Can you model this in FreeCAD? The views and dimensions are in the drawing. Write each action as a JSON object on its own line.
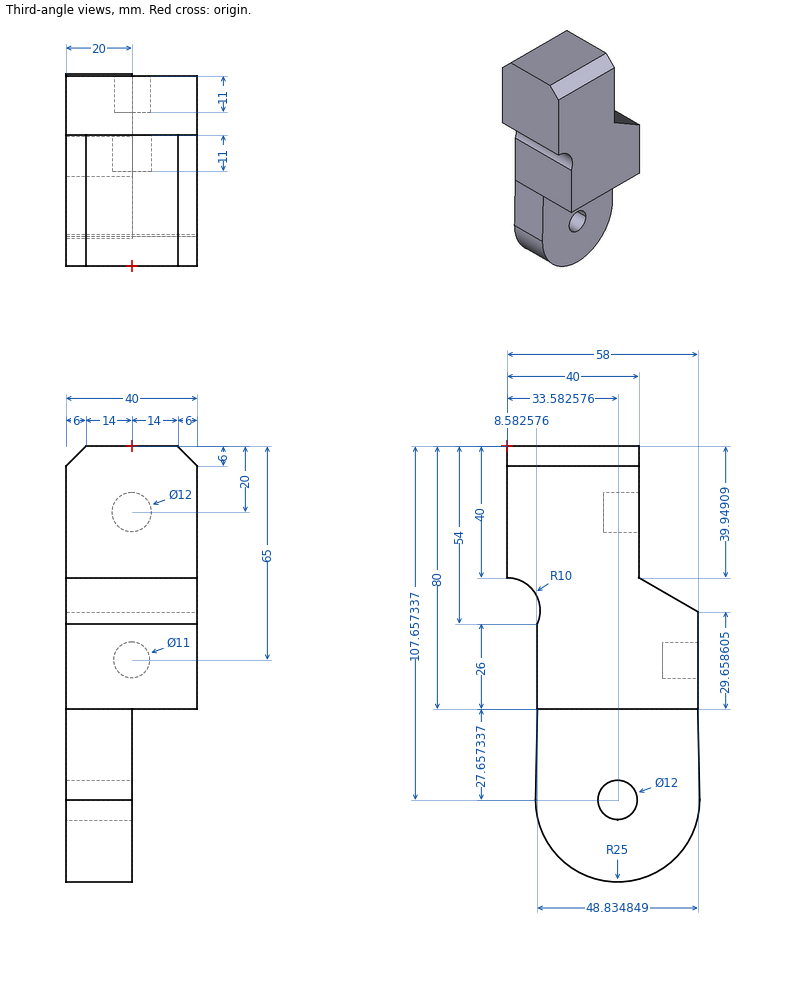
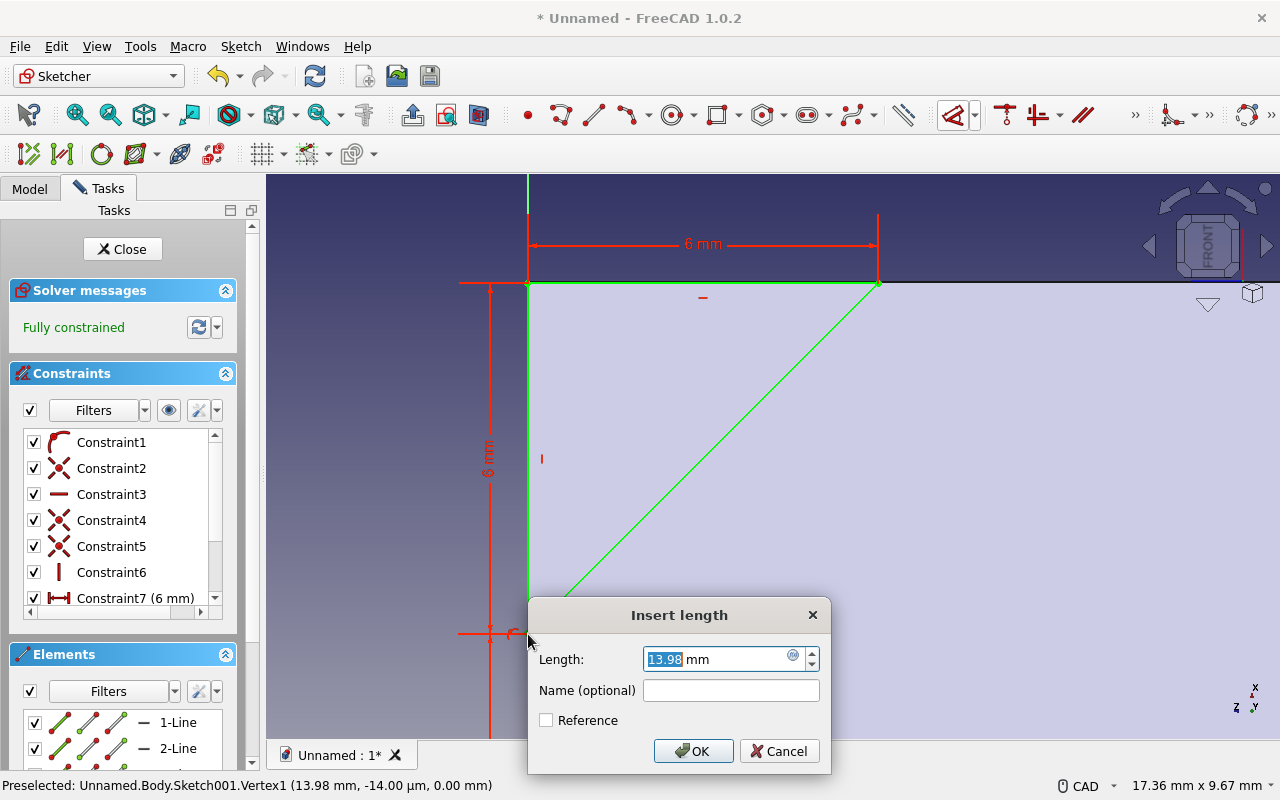
{"action": "type", "text": "14"}
{"action": "key", "text": "Return"}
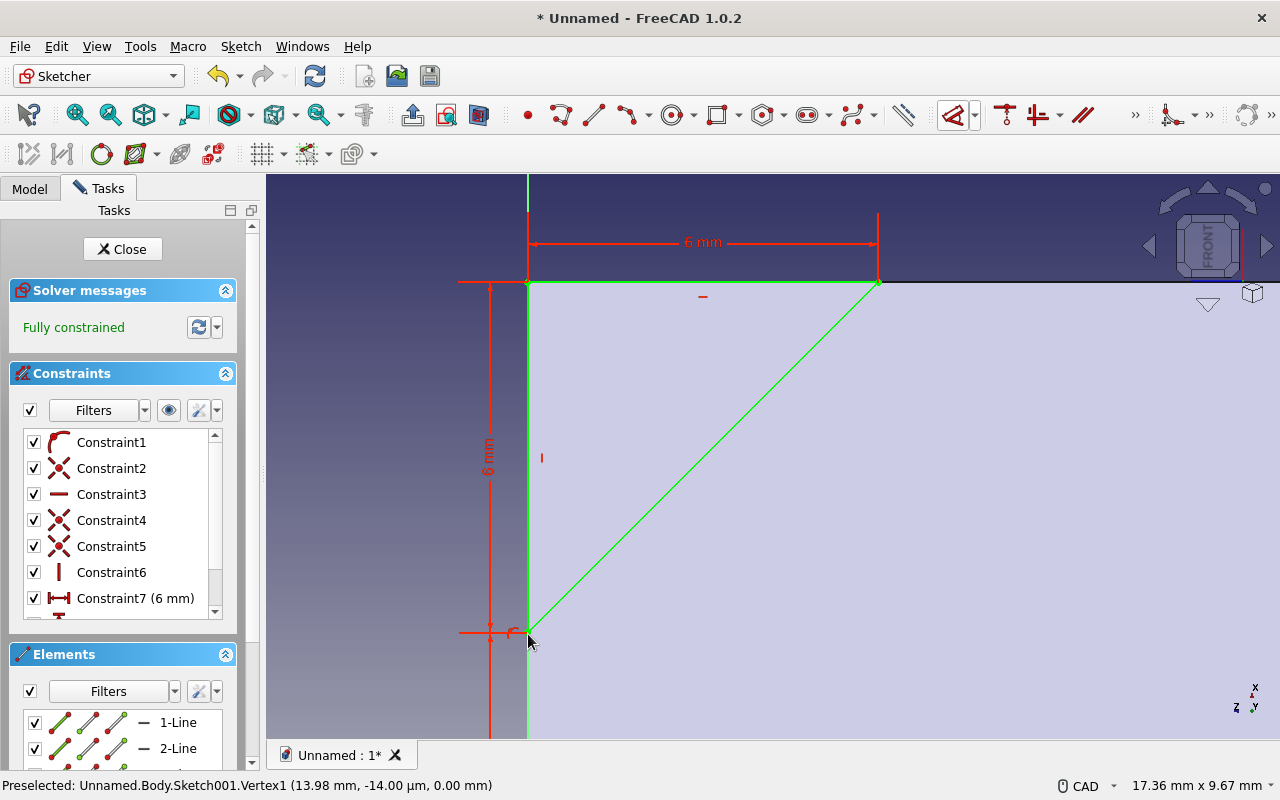
{"action": "left_click", "coordinate": [123, 249]}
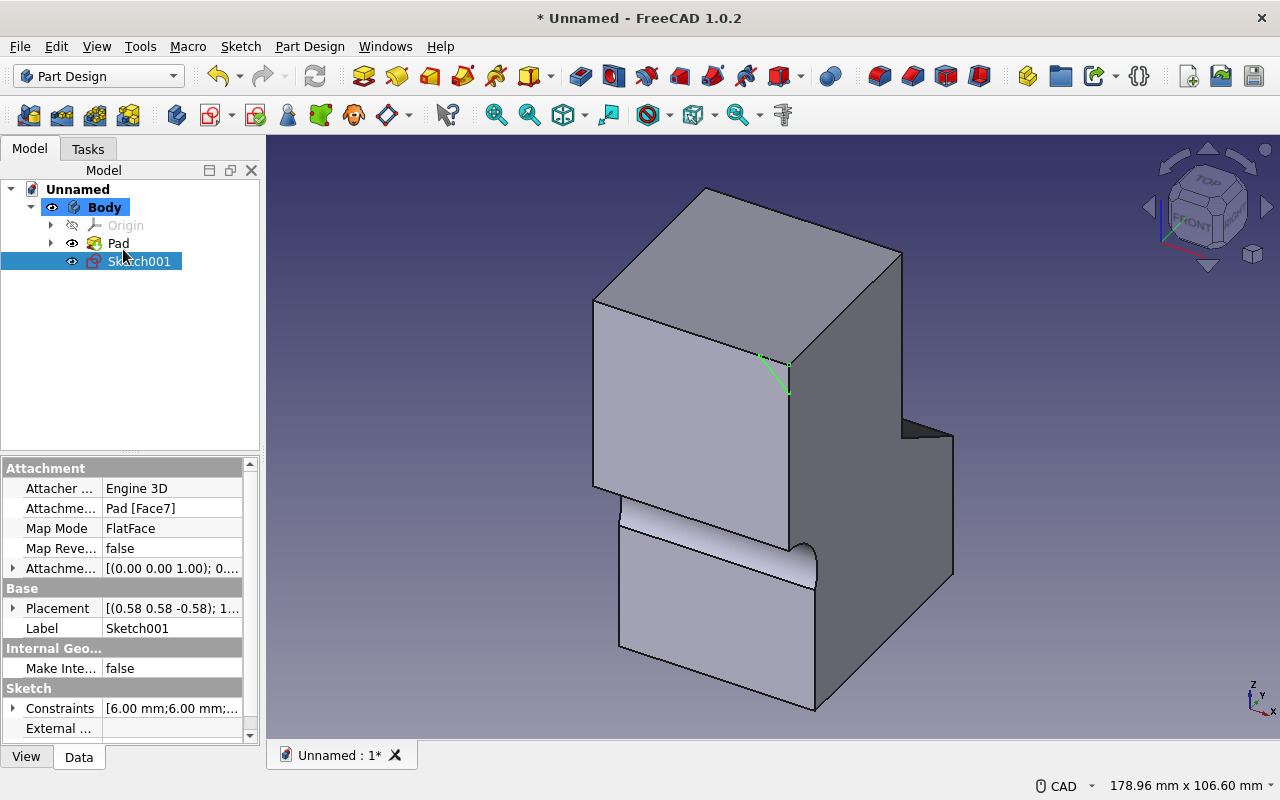
{"action": "left_click", "coordinate": [581, 76]}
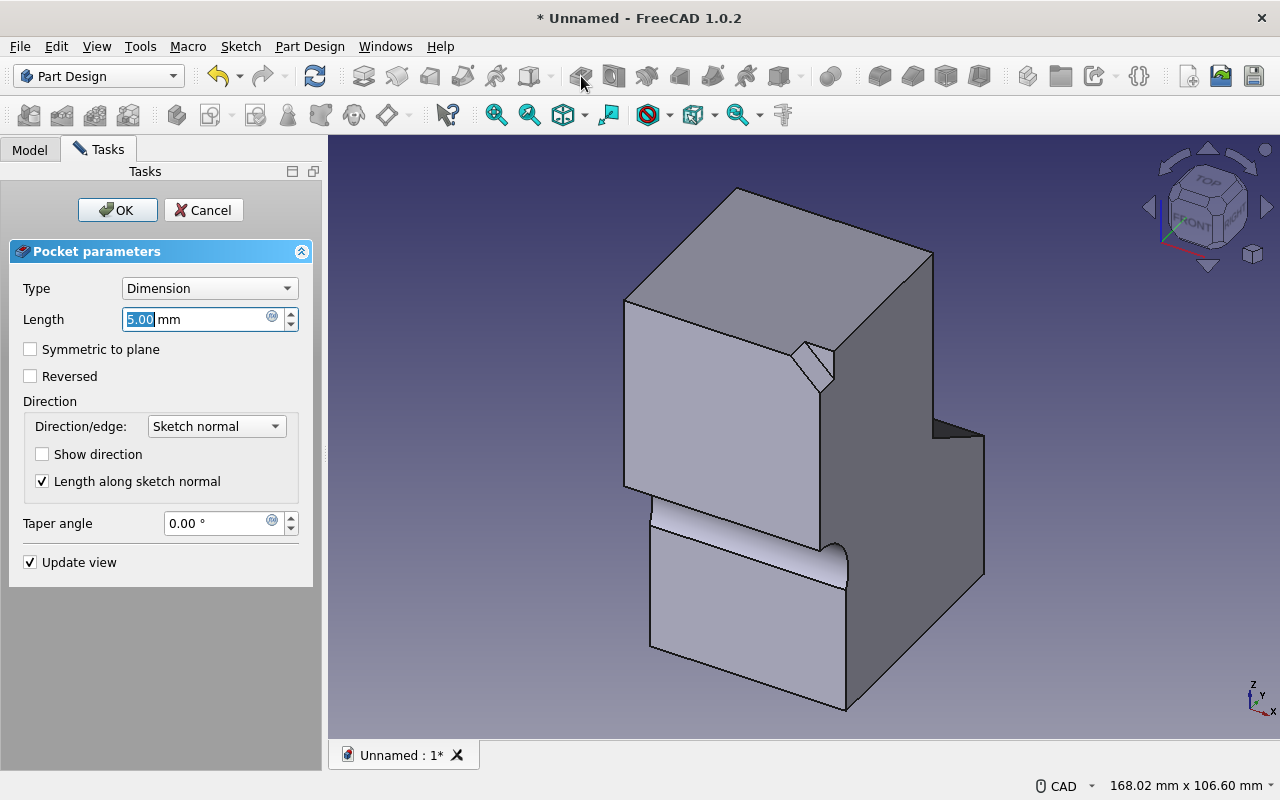
{"action": "left_click", "coordinate": [210, 288]}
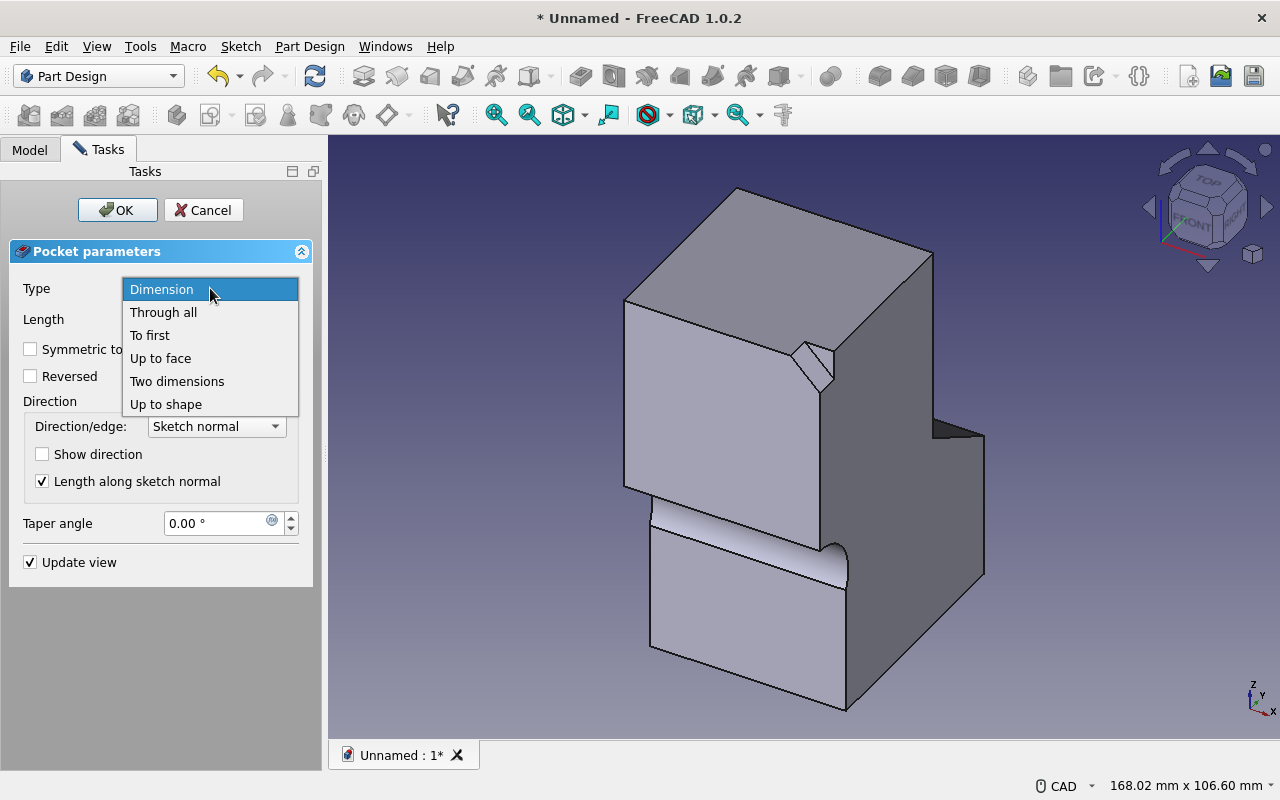
{"action": "left_click", "coordinate": [208, 312]}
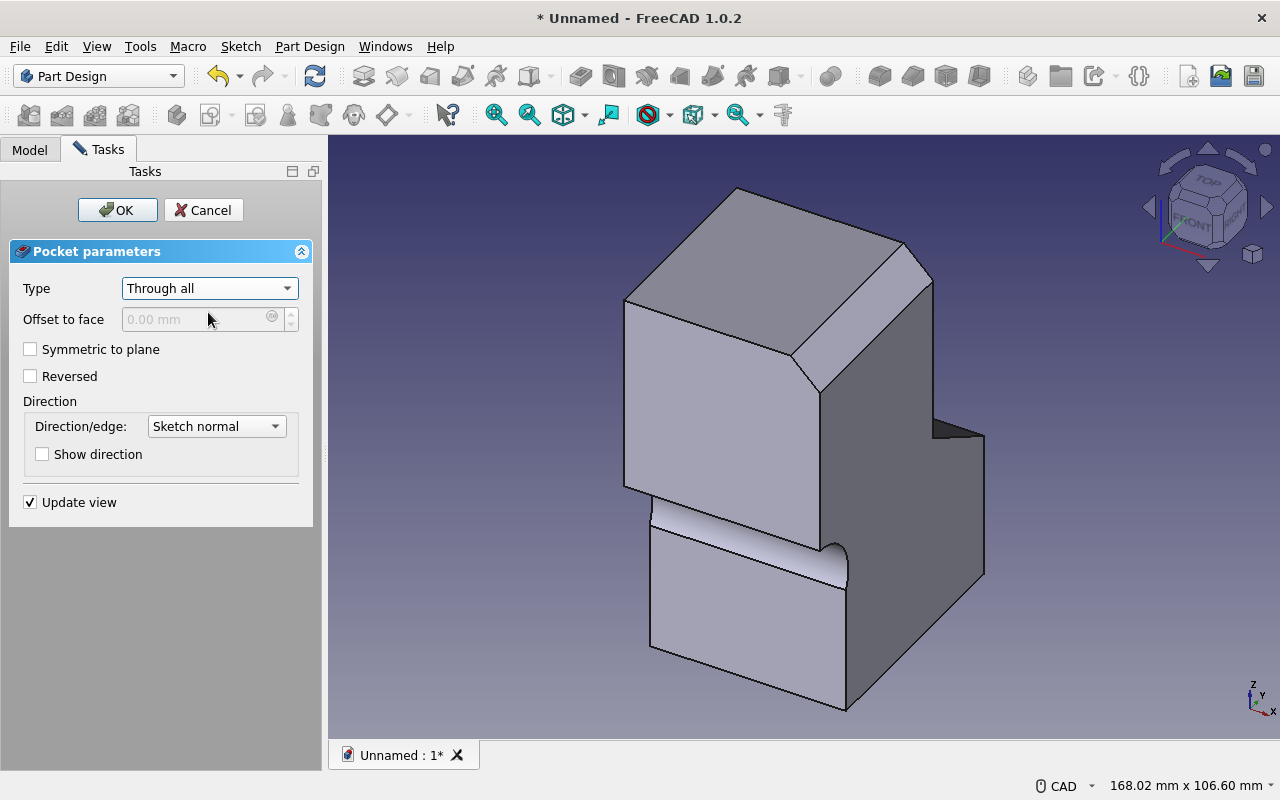
{"action": "left_click", "coordinate": [118, 210]}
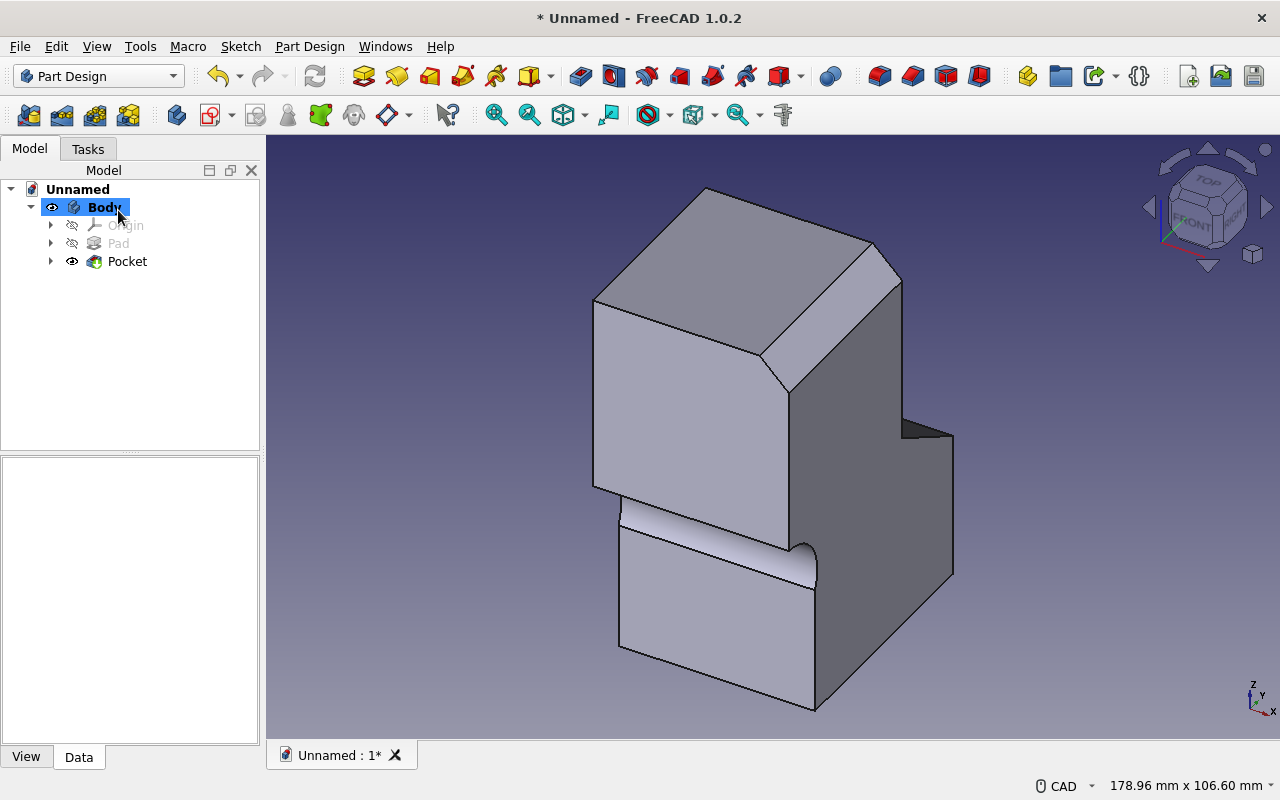
{"action": "left_click", "coordinate": [691, 425]}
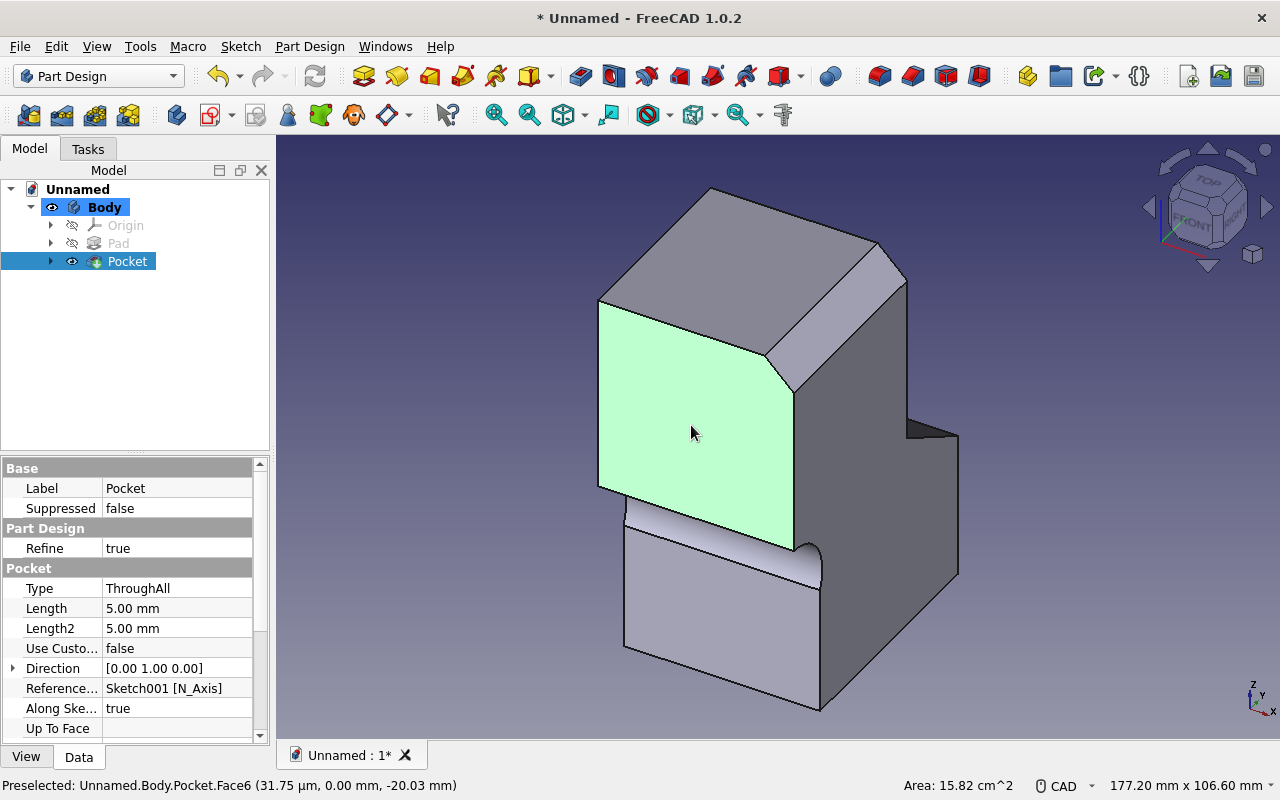
{"action": "left_click", "coordinate": [210, 116]}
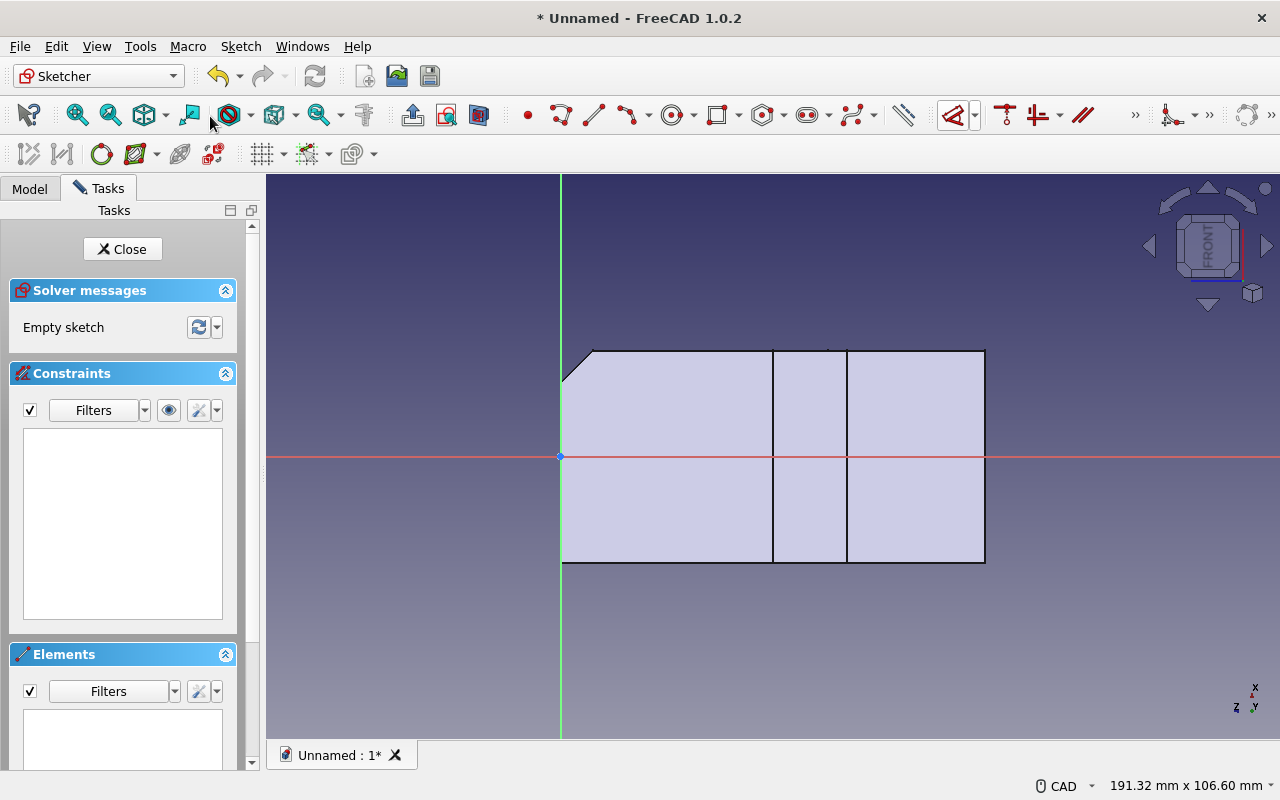
{"action": "scroll", "coordinate": [564, 556], "scroll_direction": "up", "scroll_amount": 12}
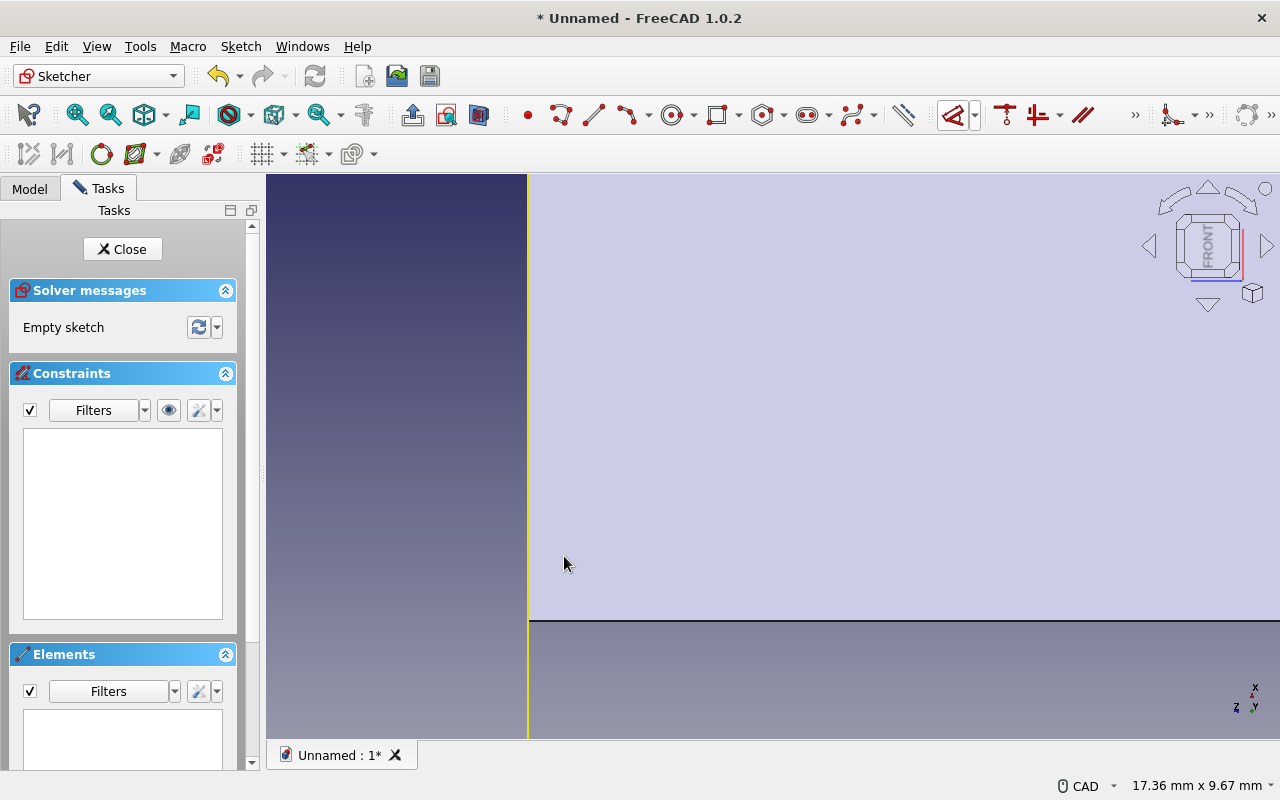
{"action": "key", "text": "g m"}